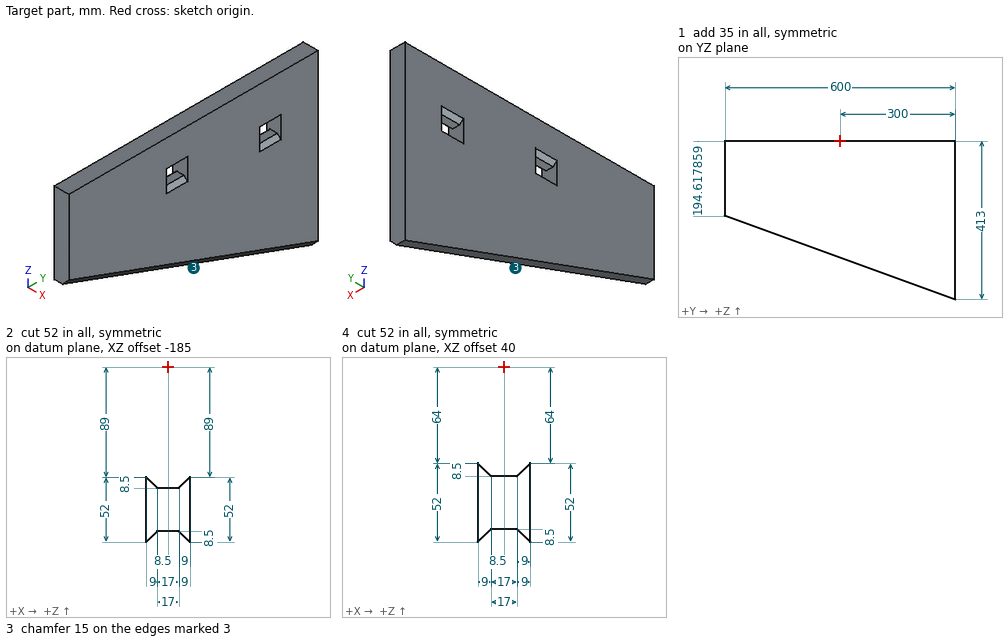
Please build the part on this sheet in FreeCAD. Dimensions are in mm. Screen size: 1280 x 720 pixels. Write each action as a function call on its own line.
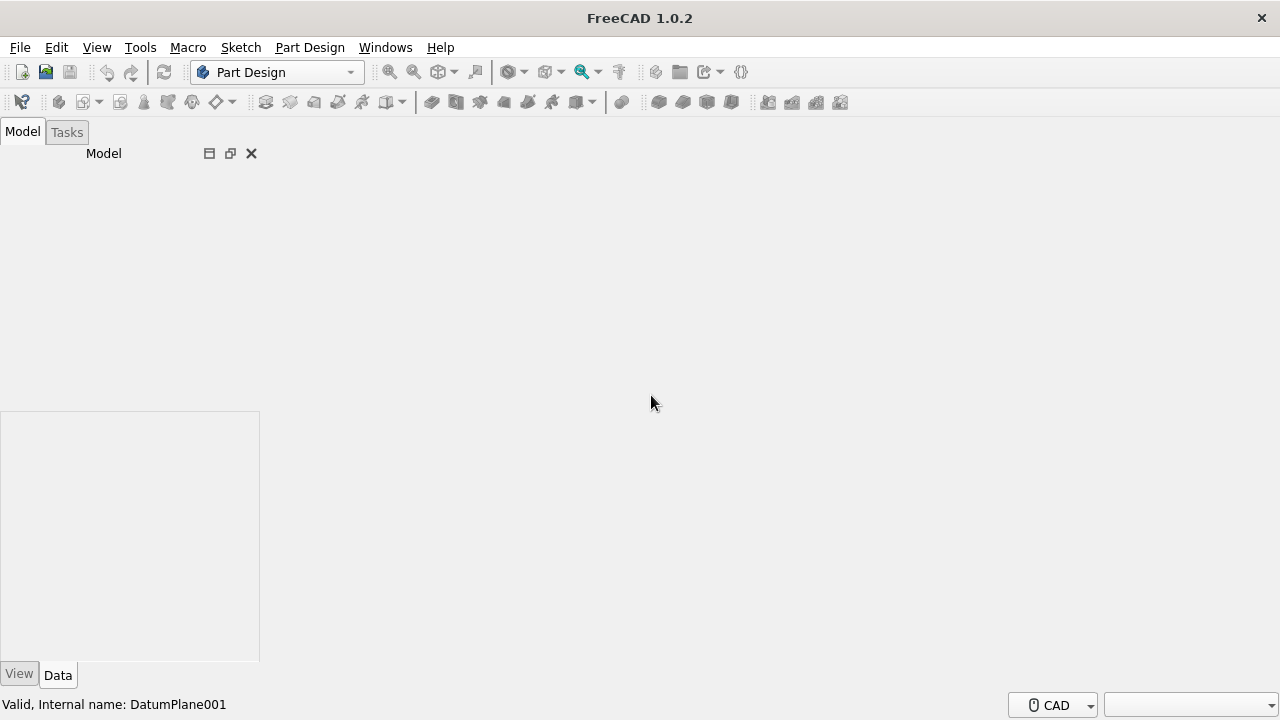
click(22, 72)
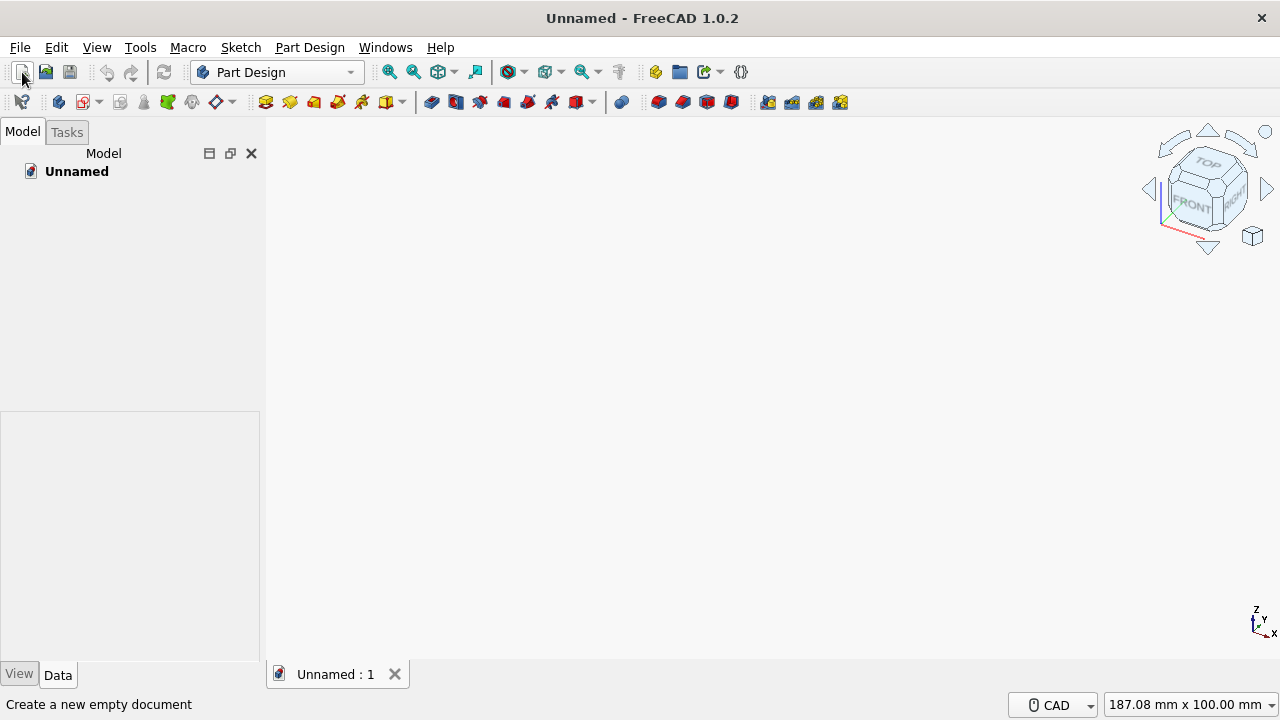
click(84, 102)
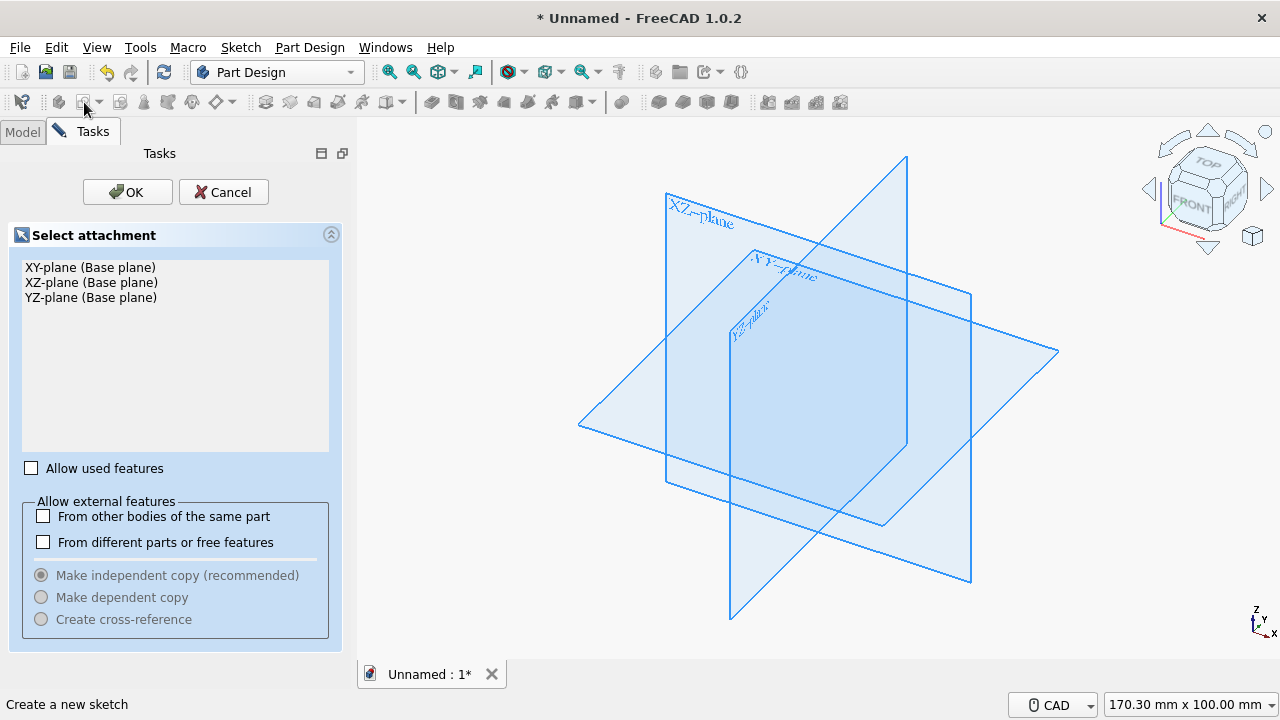
click(82, 298)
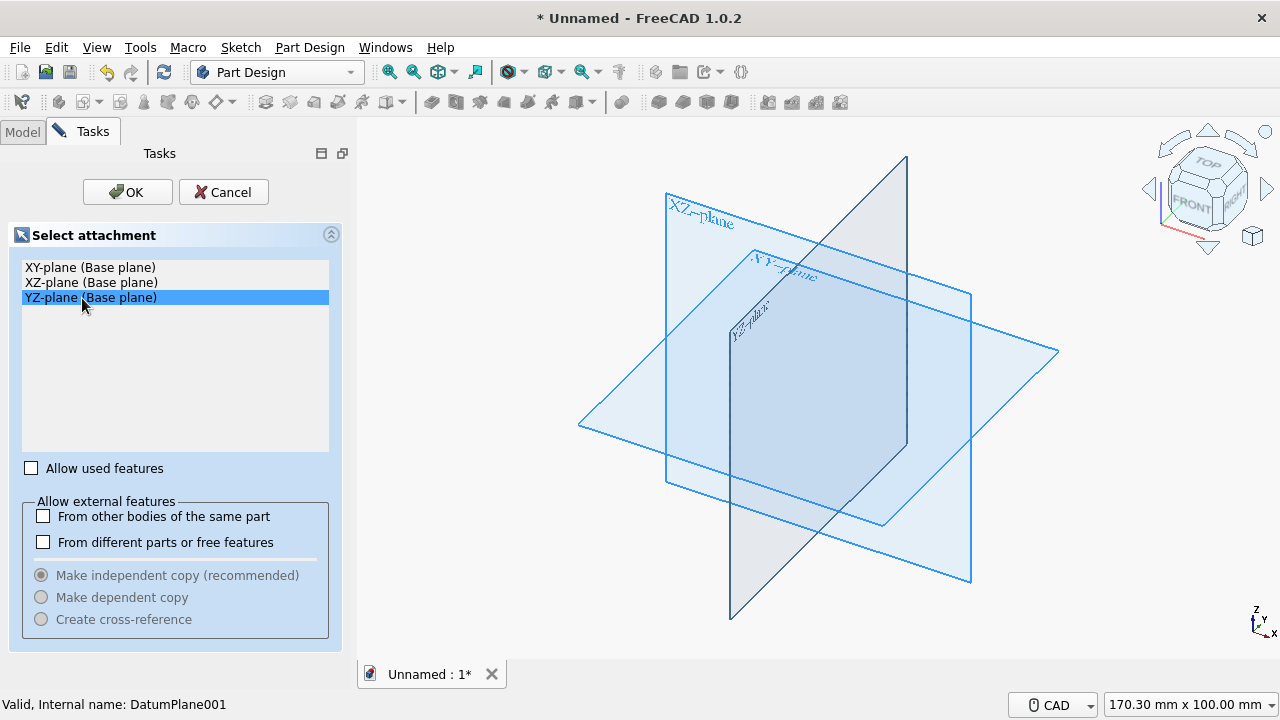
click(128, 192)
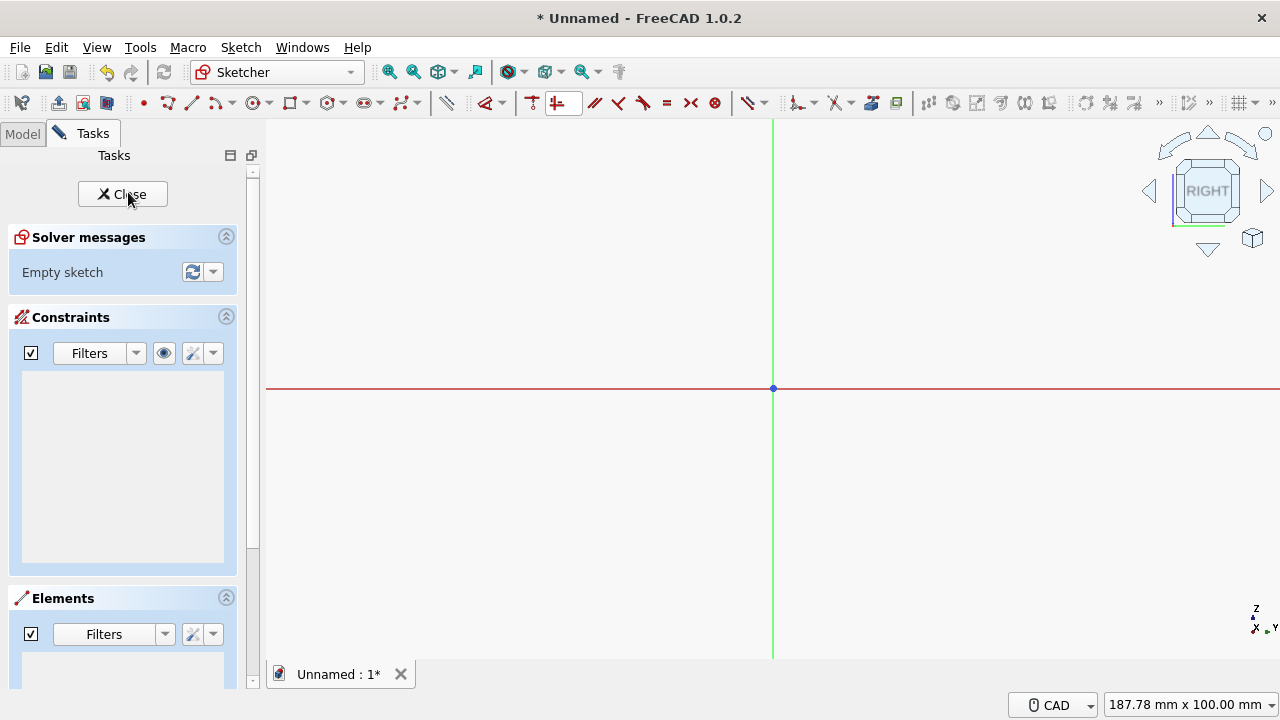
scroll(691, 168, down, 9)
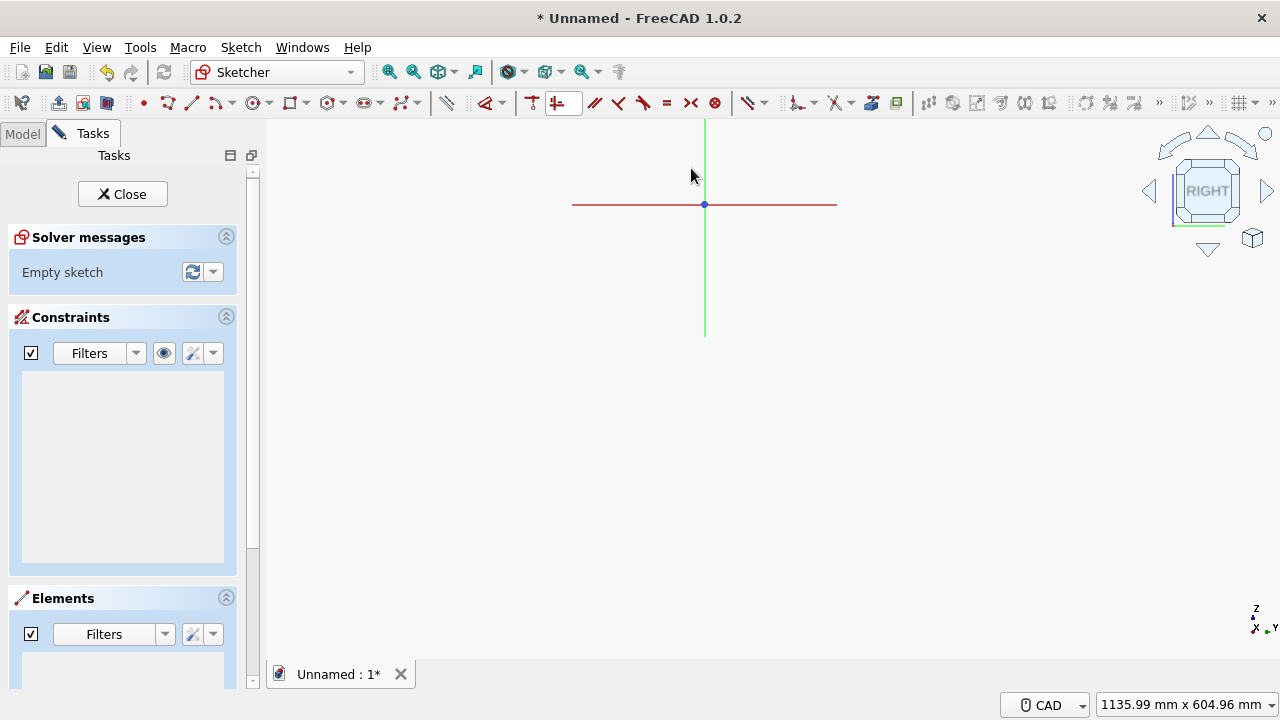
key(g)
key(m)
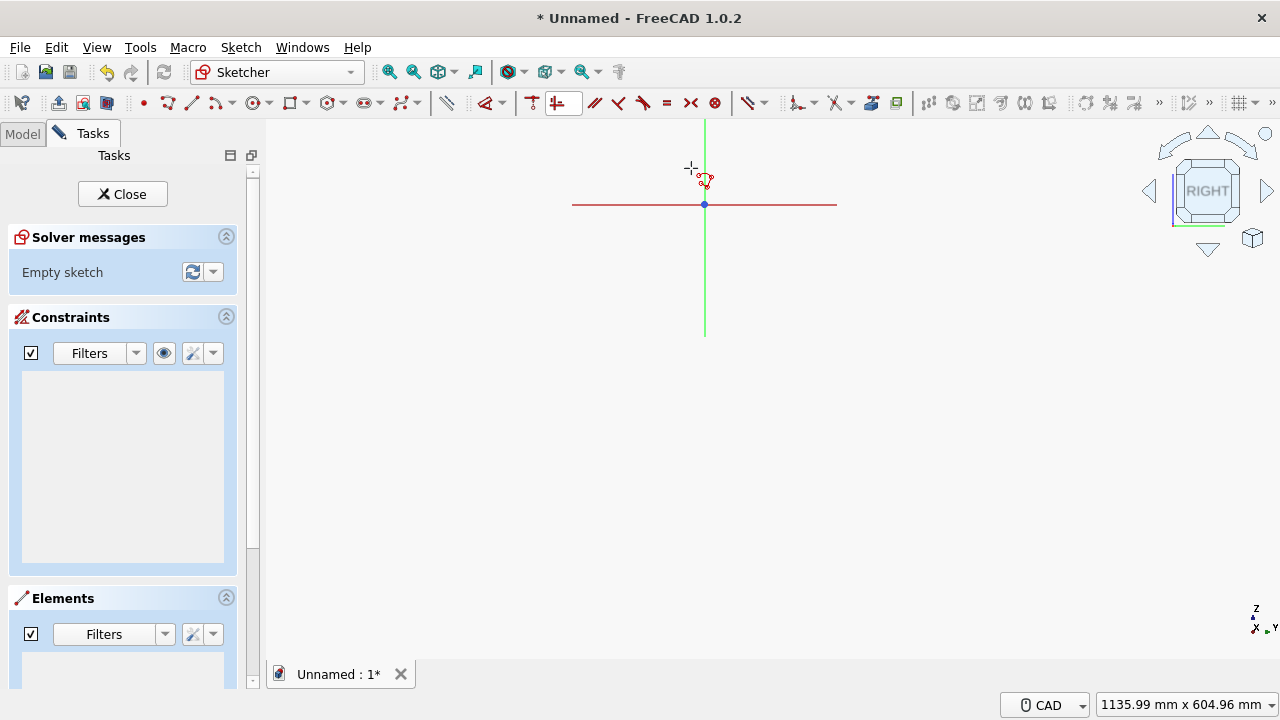
click(973, 205)
click(437, 214)
click(437, 378)
click(973, 573)
click(973, 206)
key(Escape)
key(Escape)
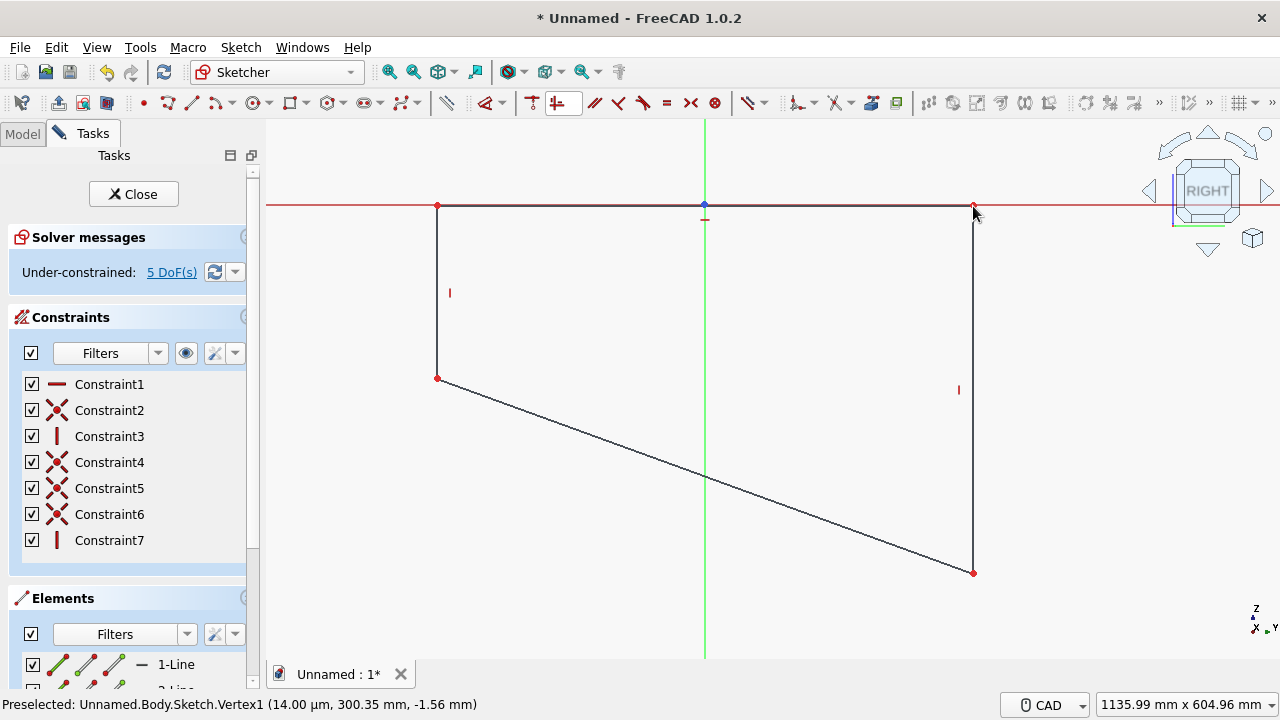
click(973, 206)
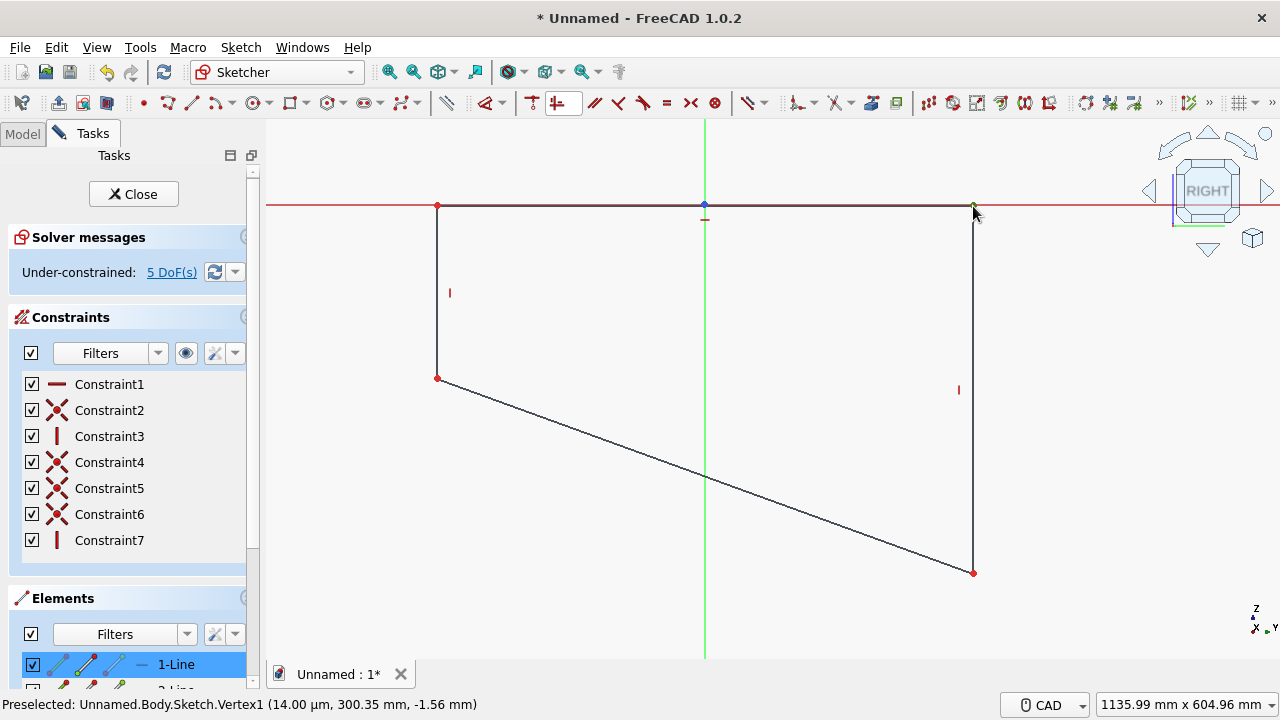
click(353, 205)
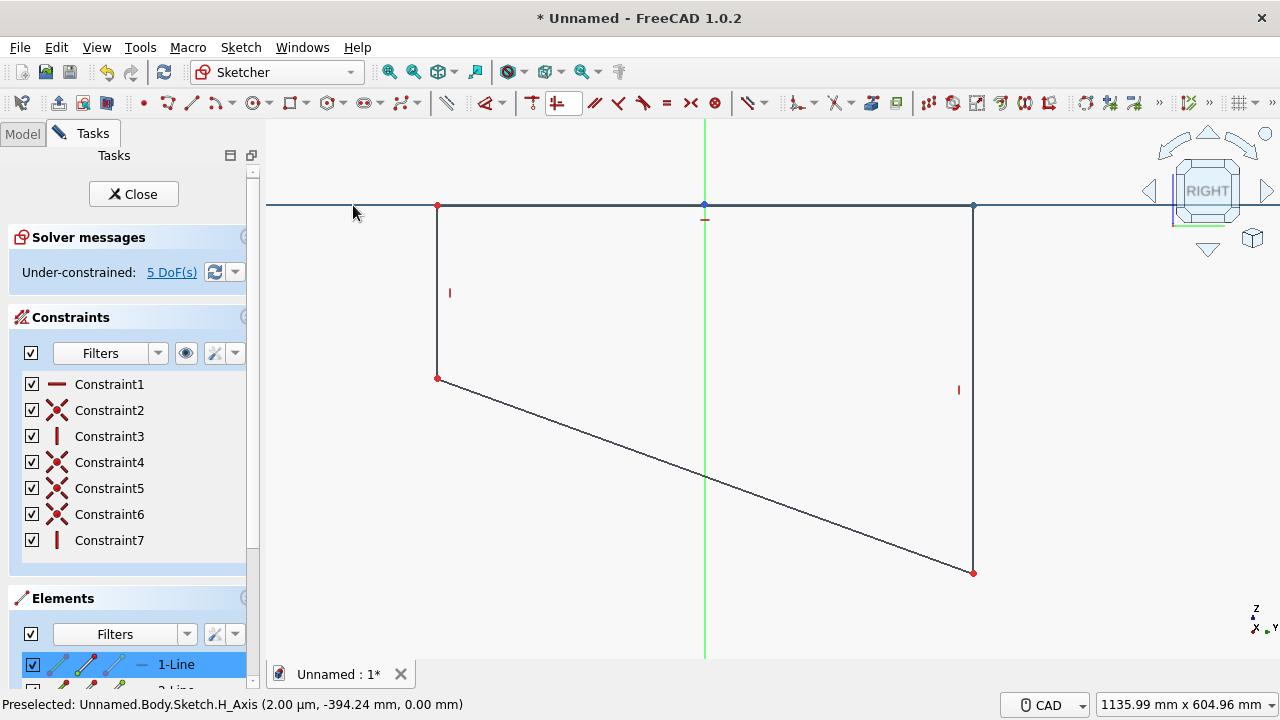
click(532, 104)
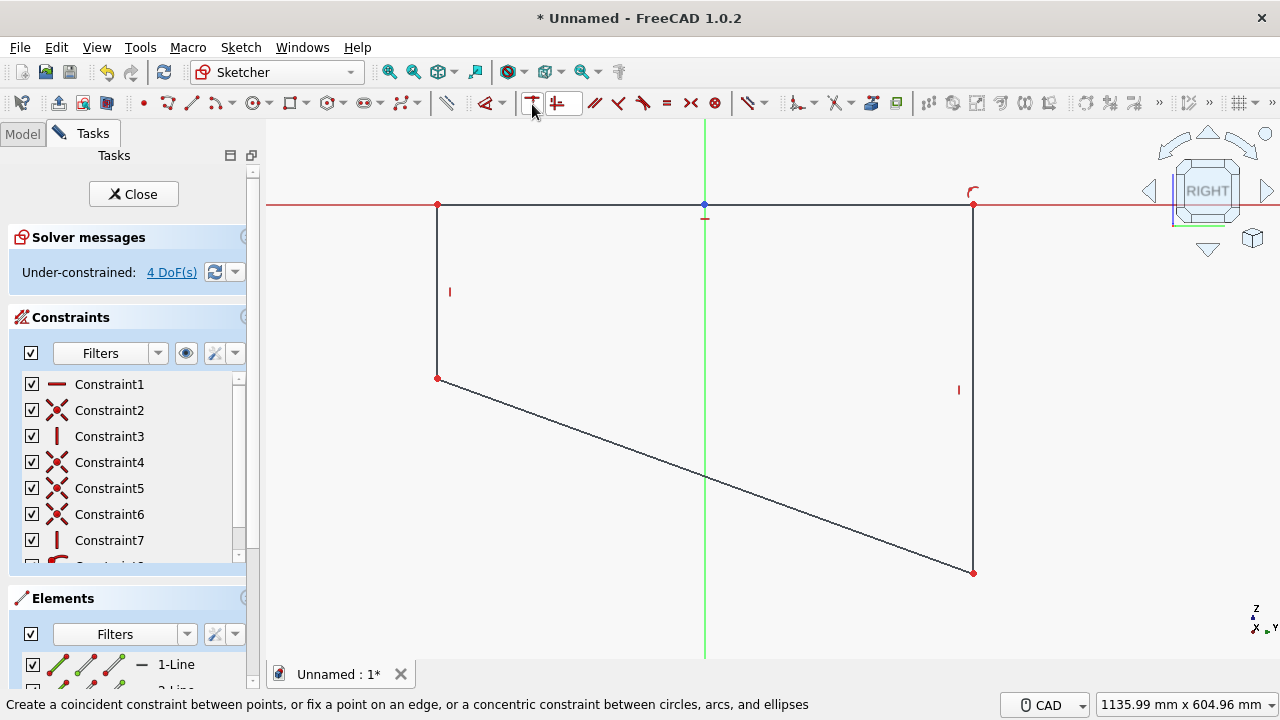
click(812, 205)